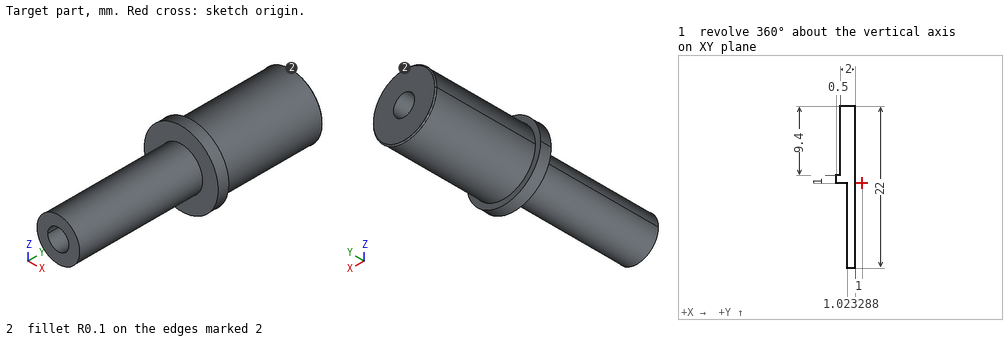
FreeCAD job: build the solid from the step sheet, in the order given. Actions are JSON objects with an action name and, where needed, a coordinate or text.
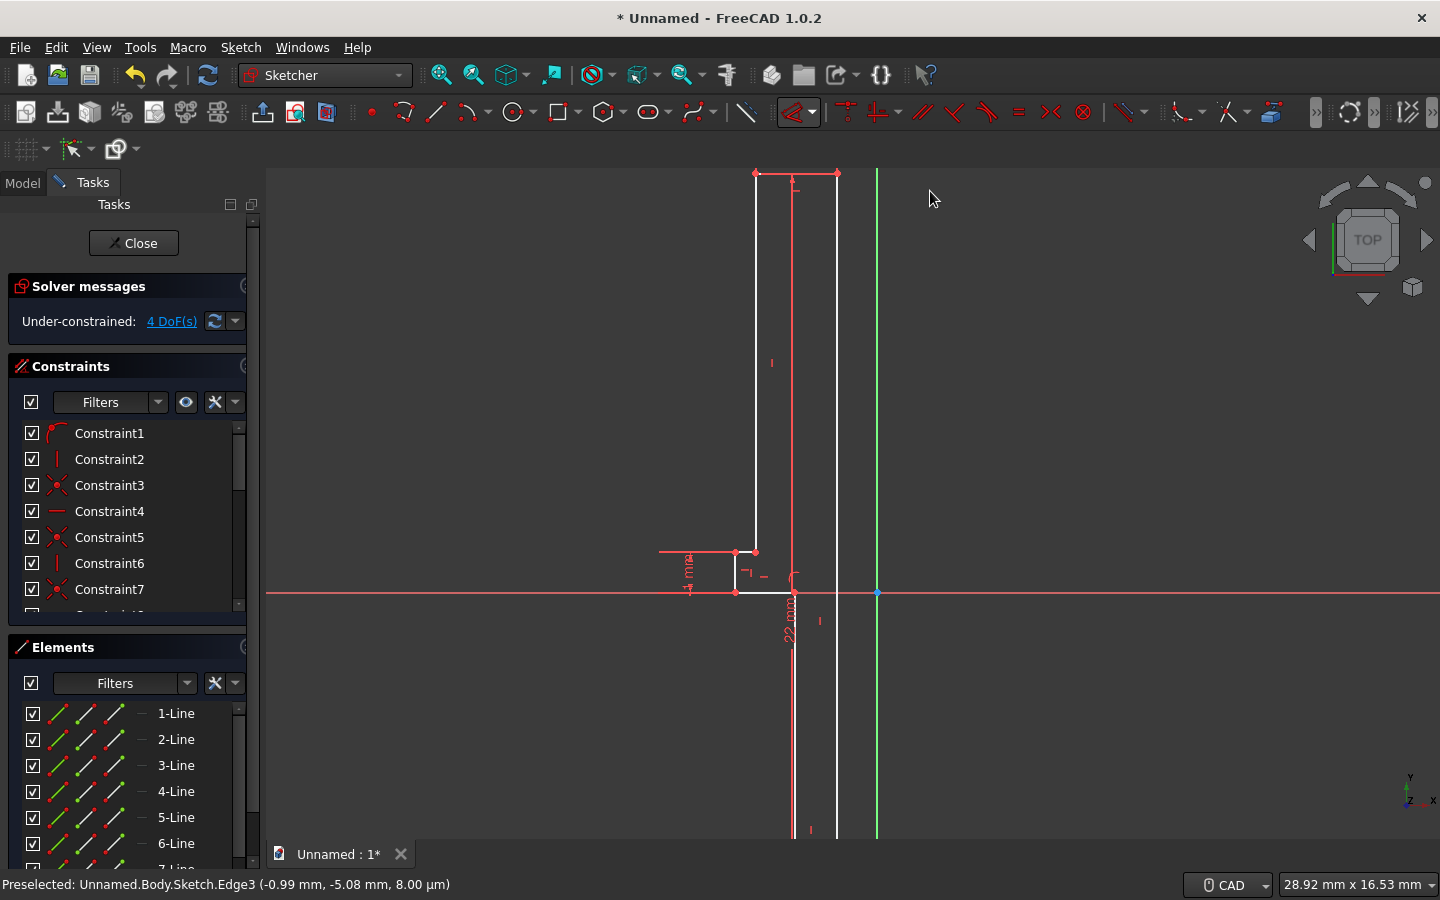
{"action": "scroll", "coordinate": [767, 411], "scroll_direction": "down", "scroll_amount": 4}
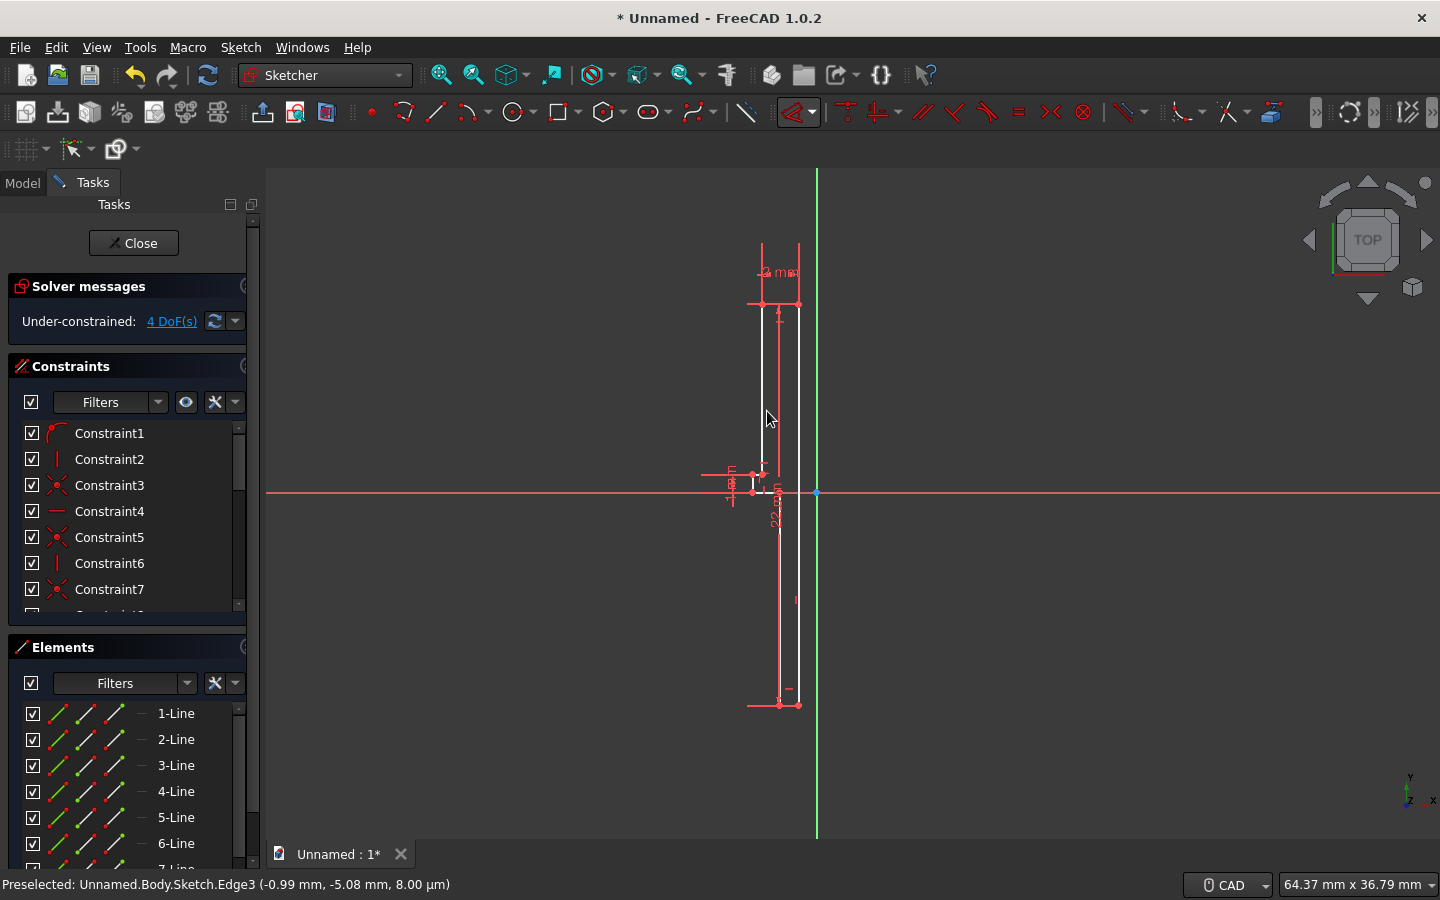
{"action": "scroll", "coordinate": [799, 706], "scroll_direction": "up", "scroll_amount": 4}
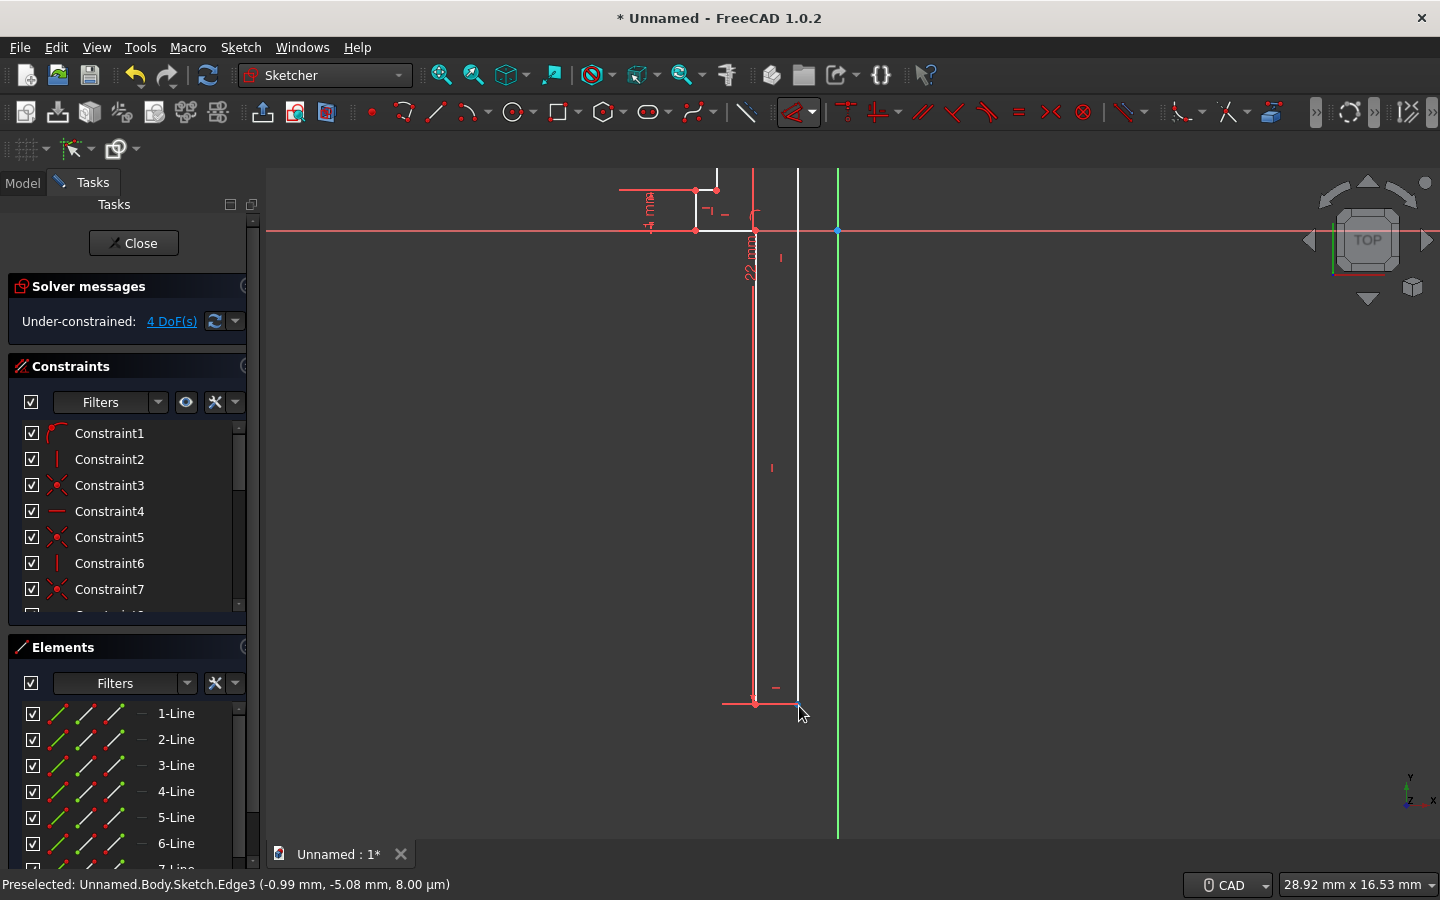
{"action": "left_click", "coordinate": [798, 704]}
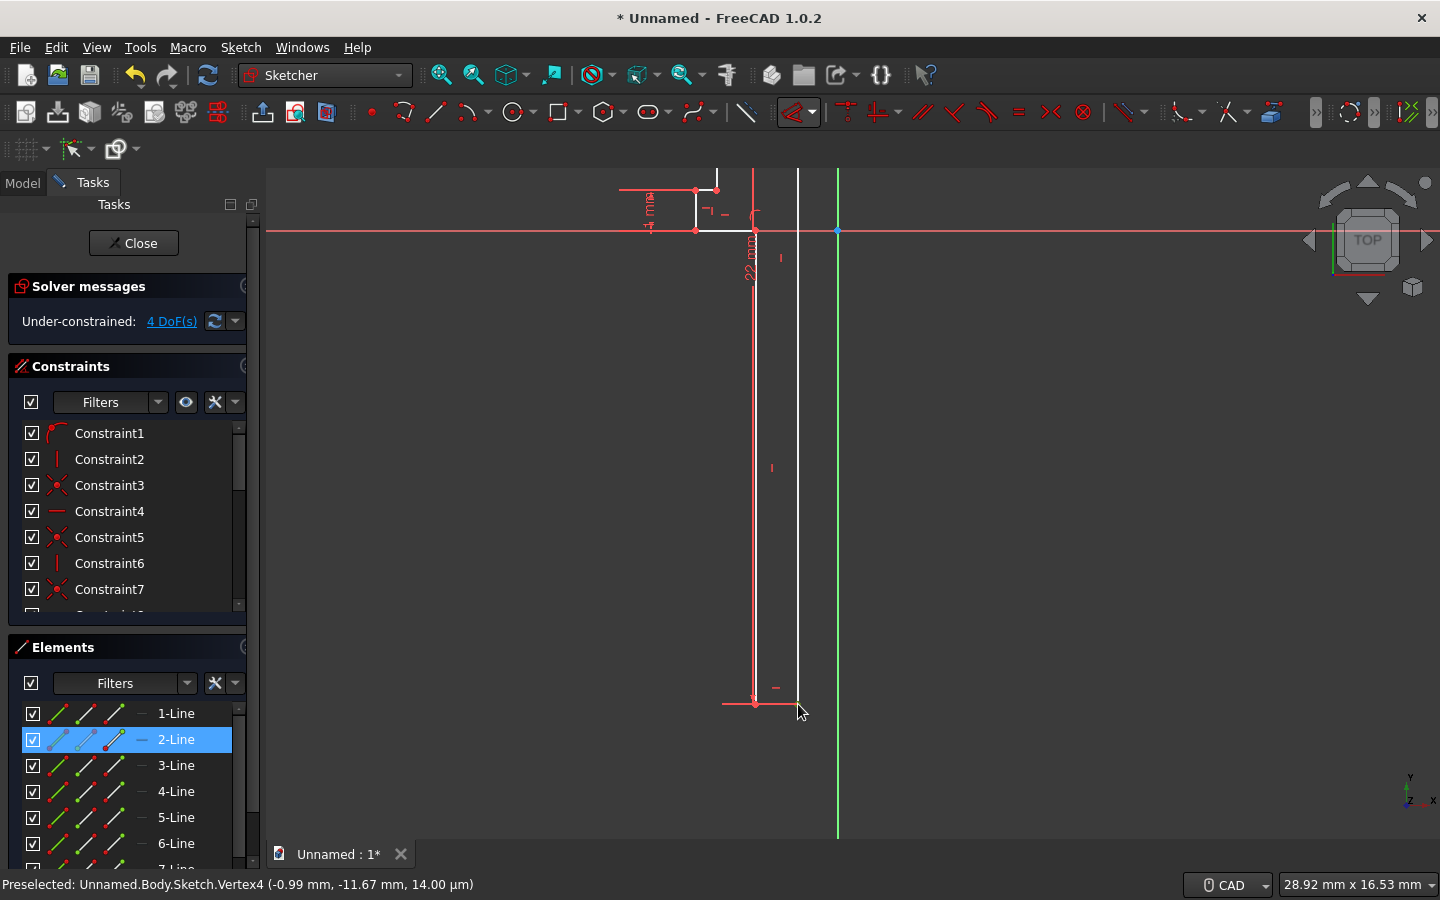
{"action": "key", "text": "l"}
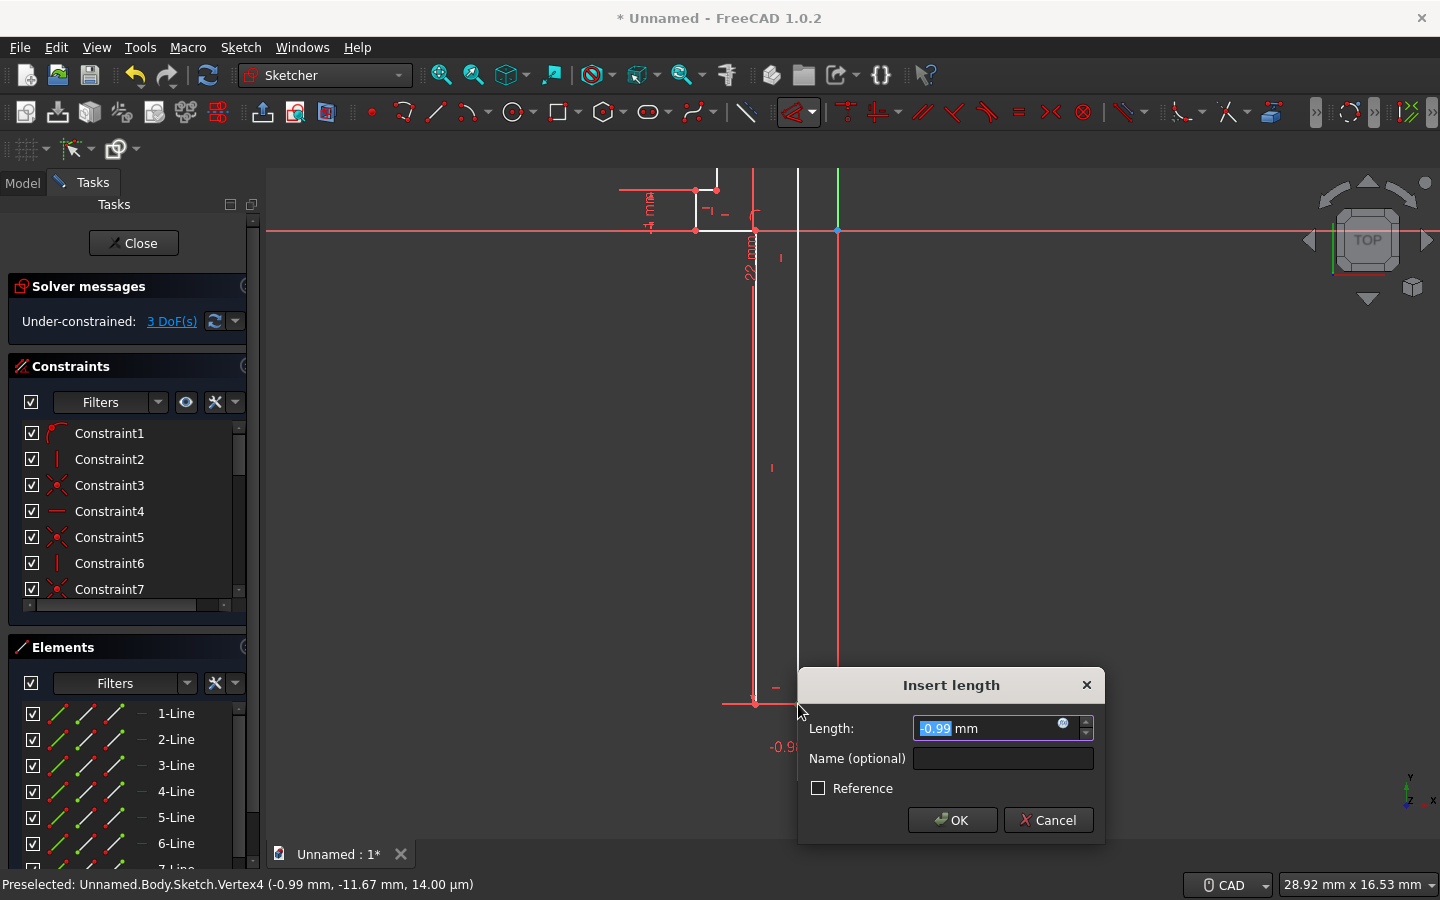
{"action": "type", "text": "-1"}
{"action": "key", "text": "Return"}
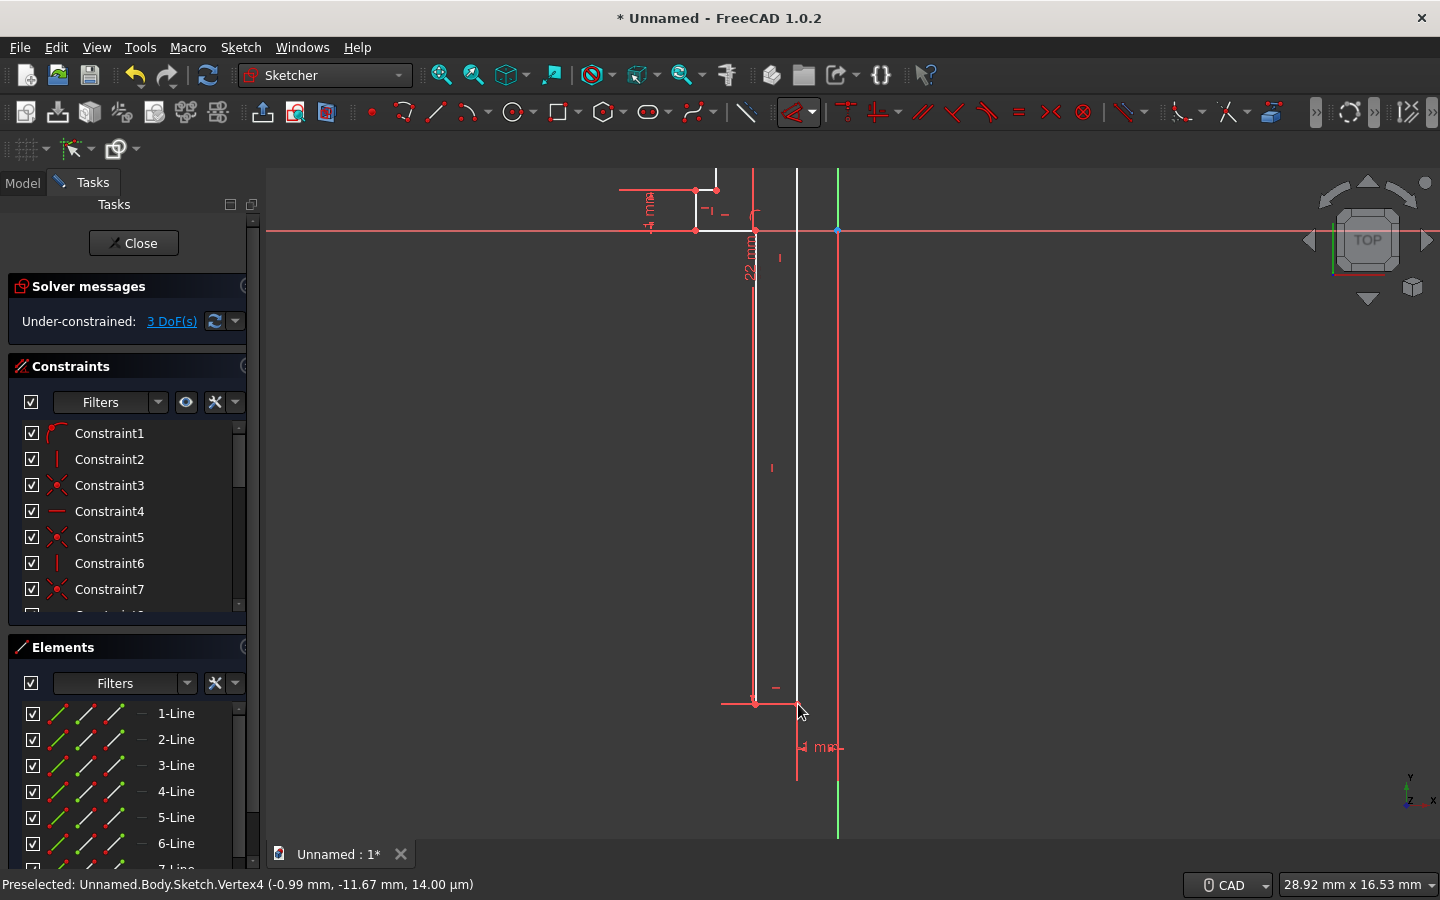
{"action": "scroll", "coordinate": [799, 706], "scroll_direction": "down", "scroll_amount": 4}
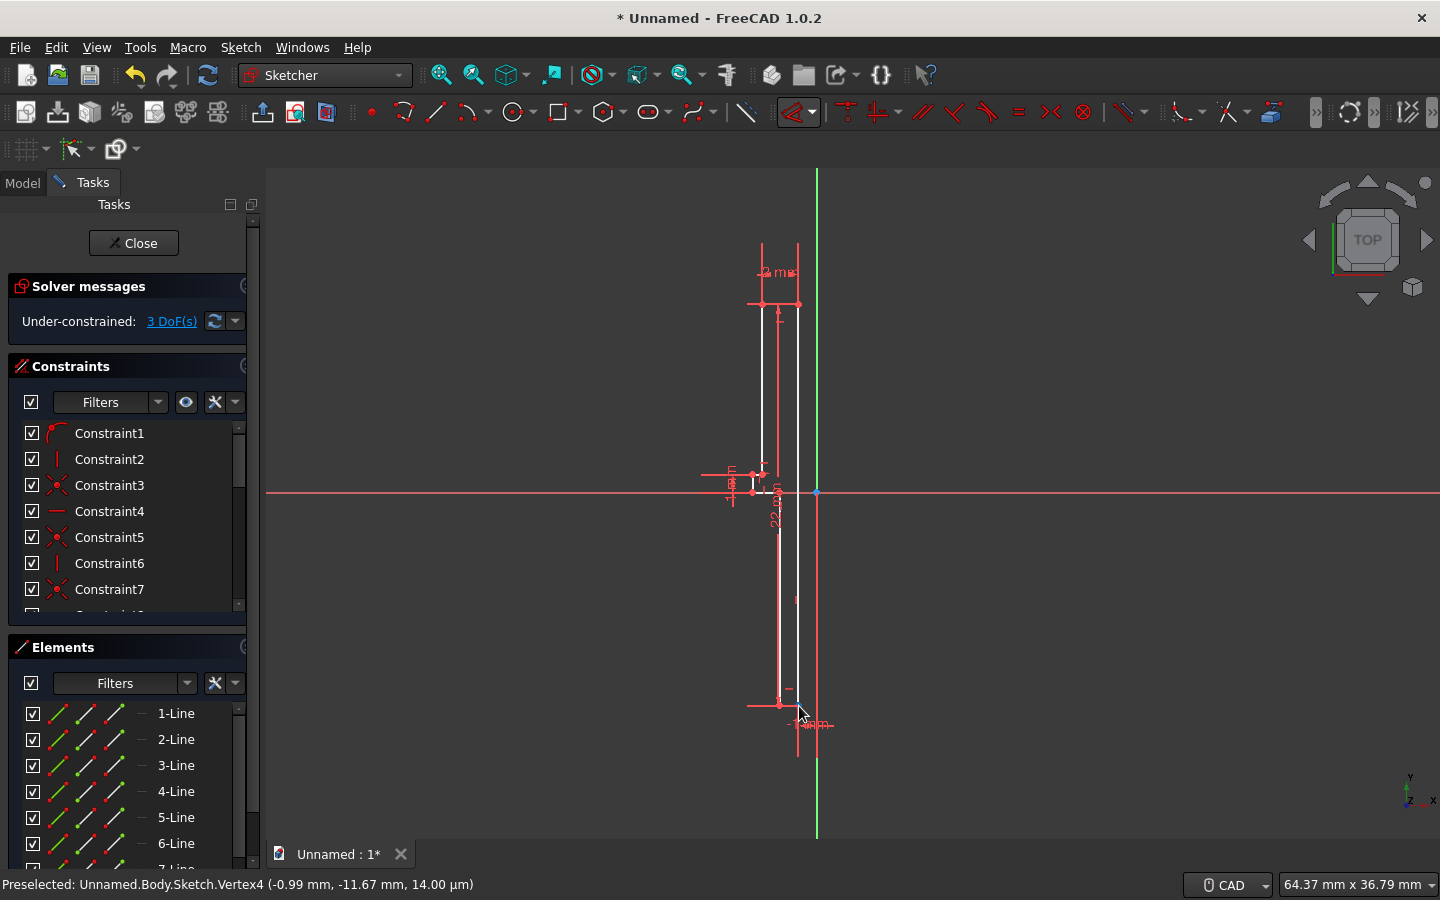
{"action": "left_click", "coordinate": [762, 356]}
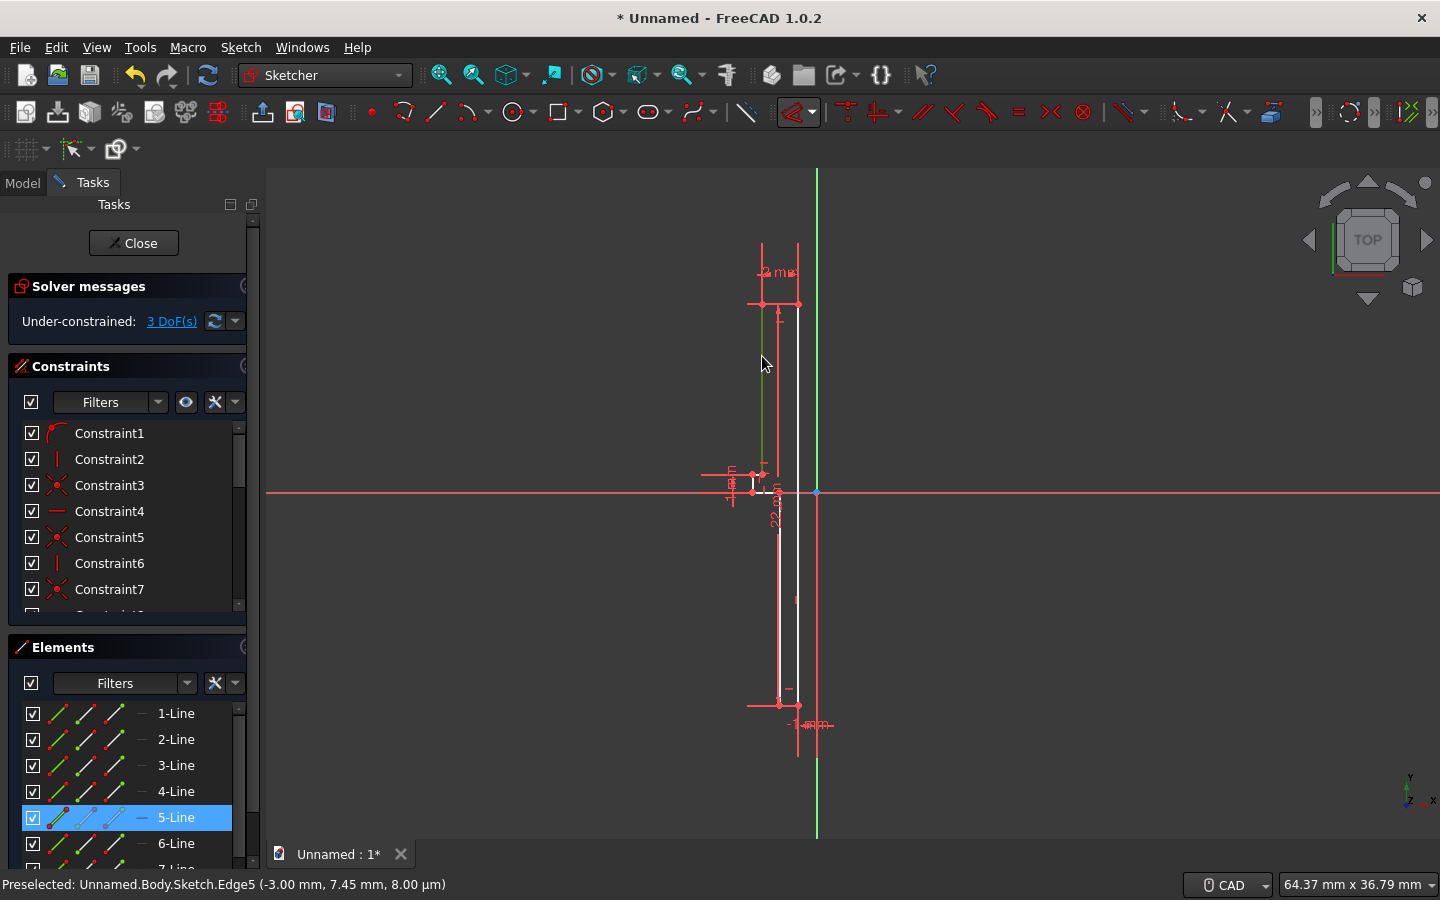
{"action": "left_click", "coordinate": [814, 112]}